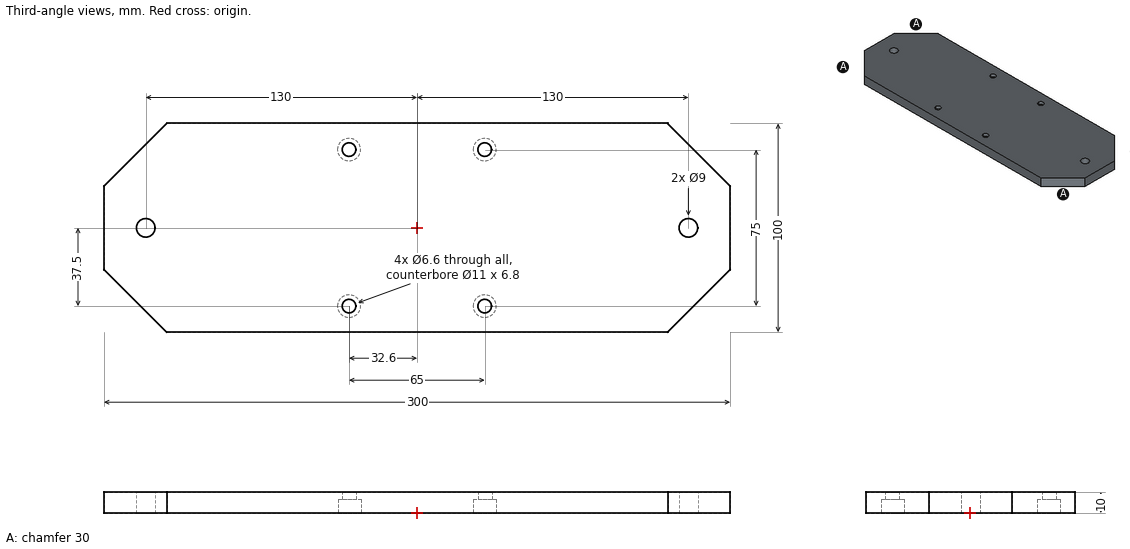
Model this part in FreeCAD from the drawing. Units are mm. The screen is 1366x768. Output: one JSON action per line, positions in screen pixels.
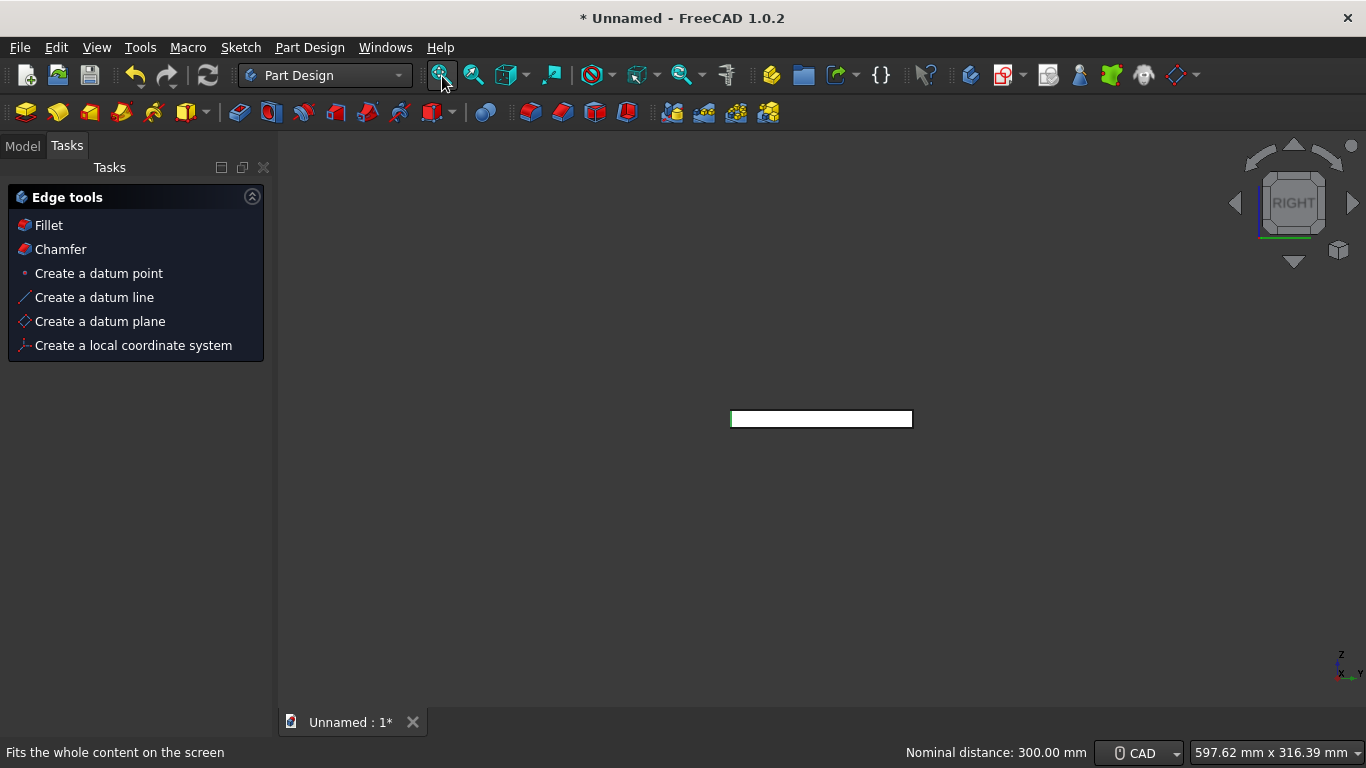
{"action": "left_click", "coordinate": [442, 76]}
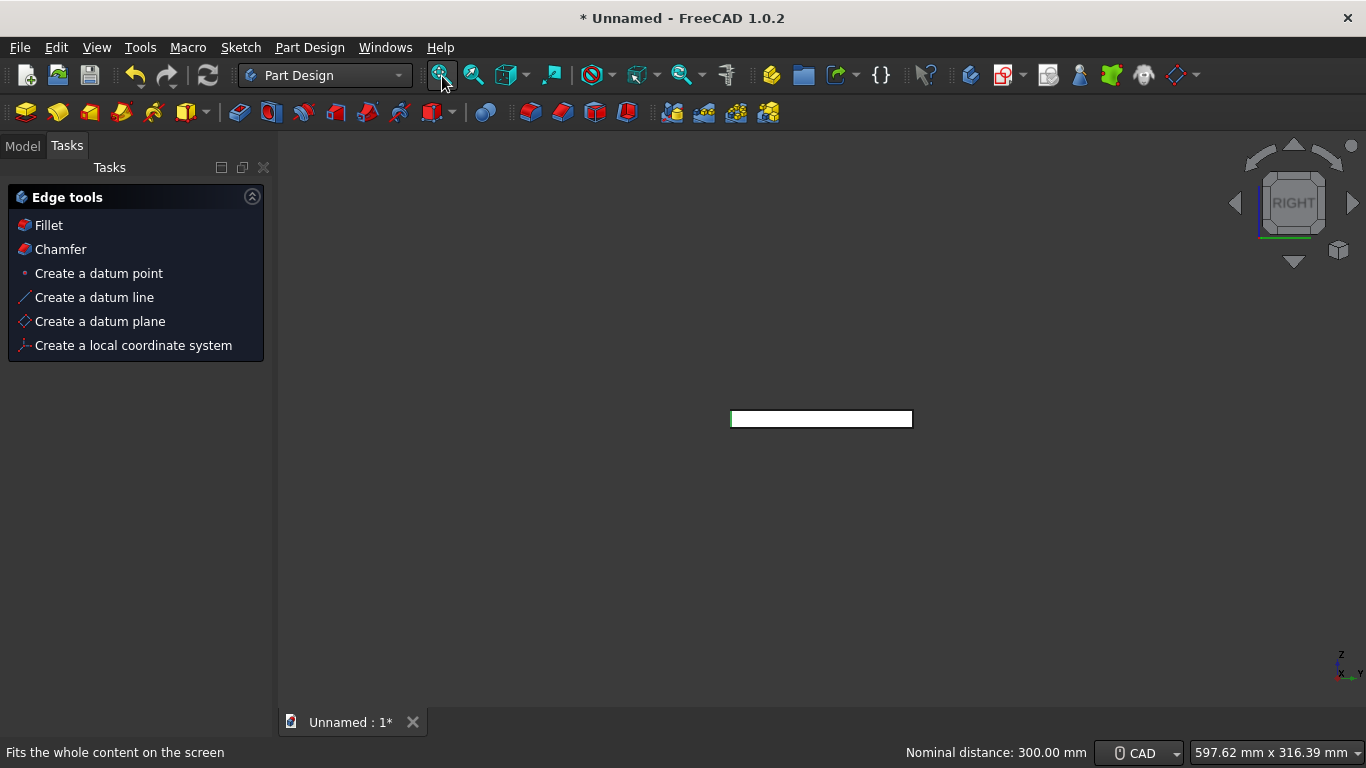
{"action": "left_click", "coordinate": [913, 418], "text": "ctrl"}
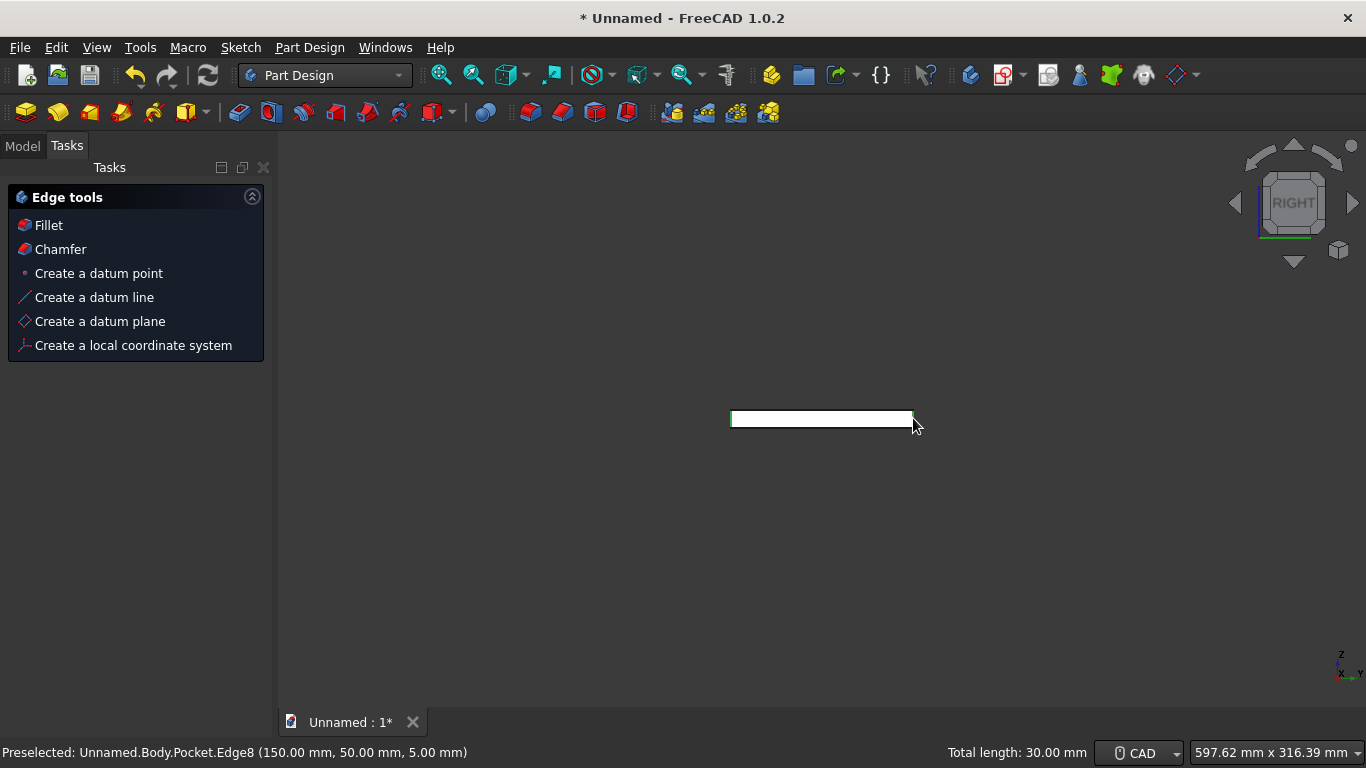
{"action": "scroll", "coordinate": [913, 418], "scroll_direction": "up", "scroll_amount": 4}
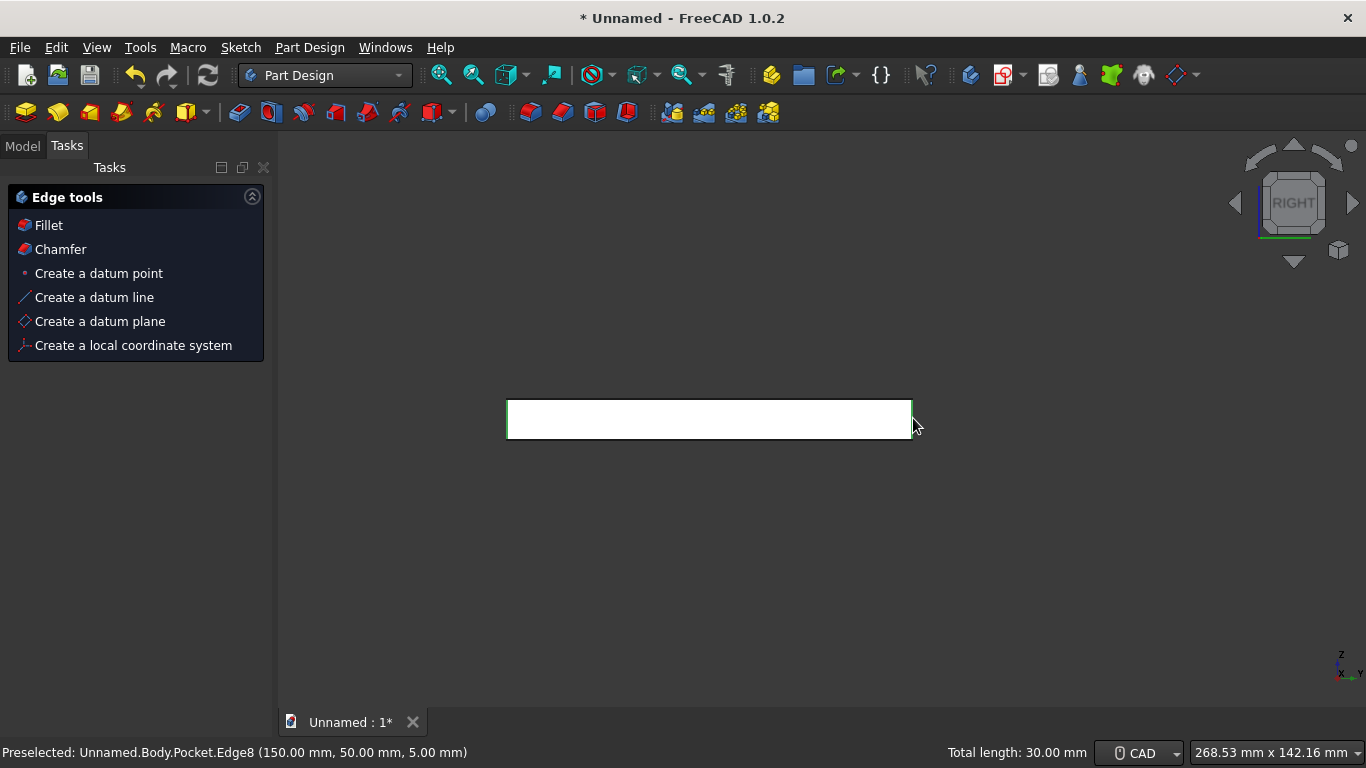
{"action": "left_click", "coordinate": [442, 76]}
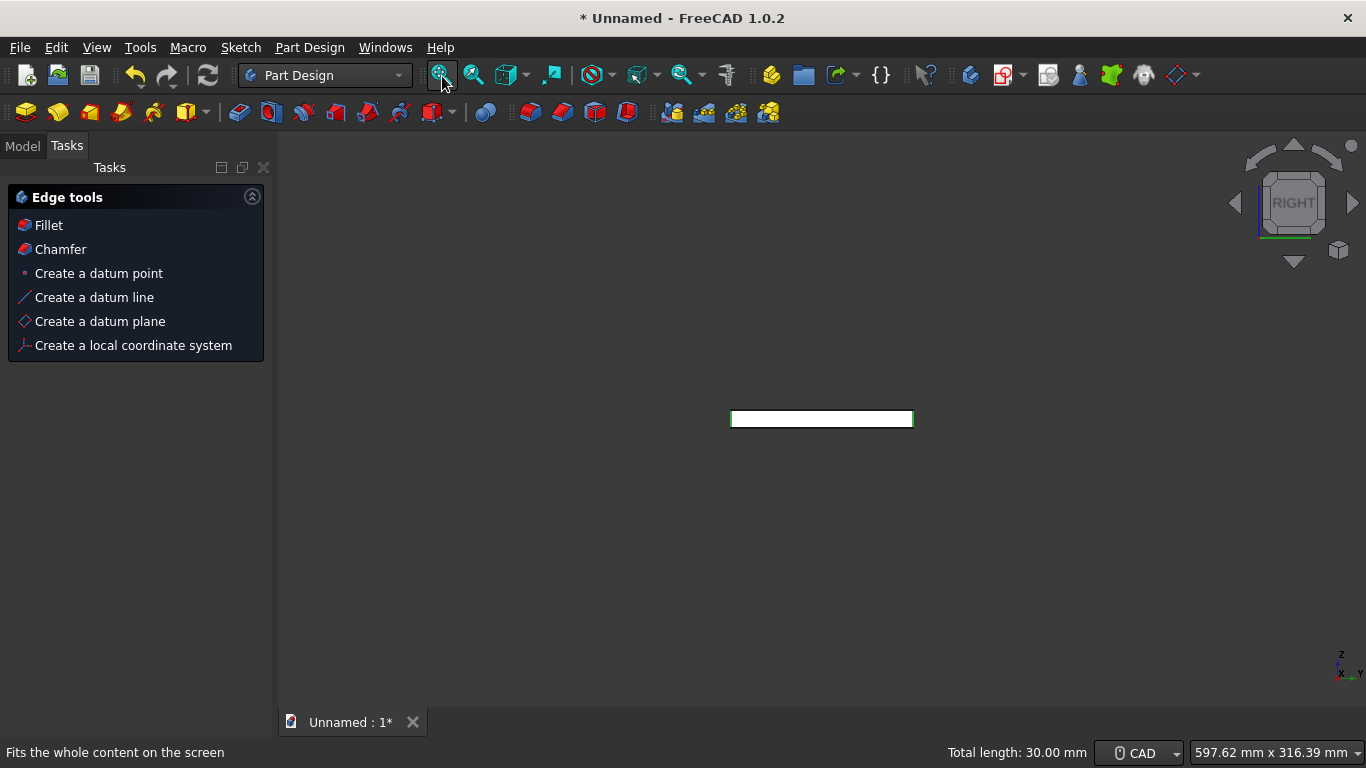
{"action": "key", "text": "5"}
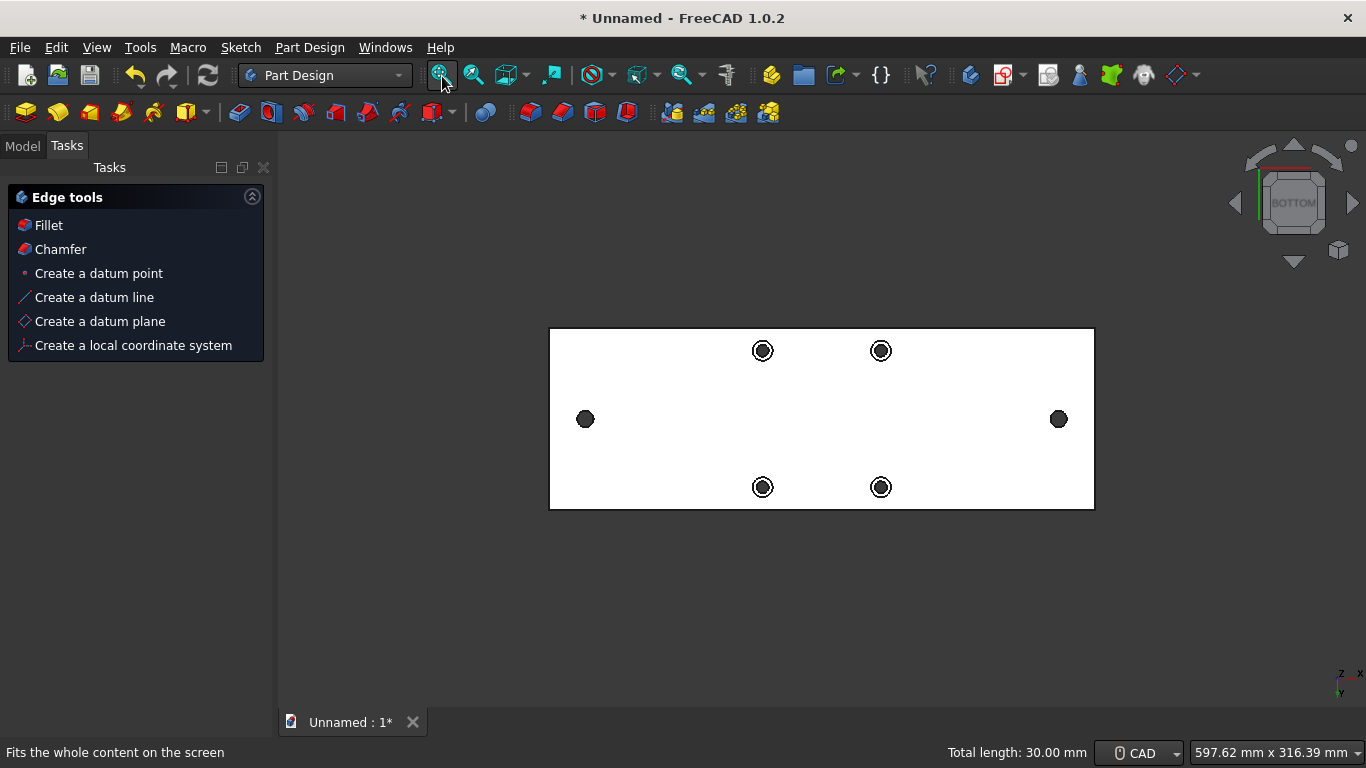
{"action": "scroll", "coordinate": [549, 509], "scroll_direction": "up", "scroll_amount": 4}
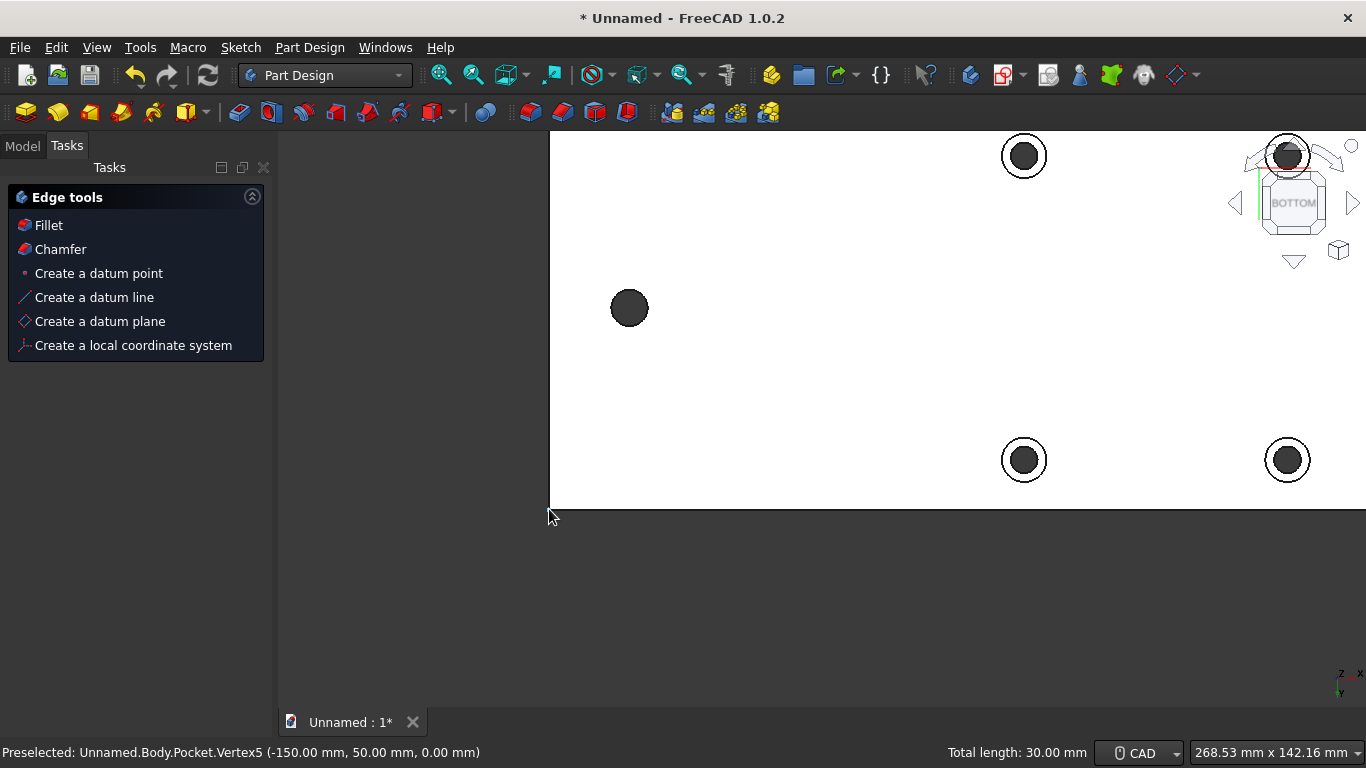
{"action": "key", "text": "v f"}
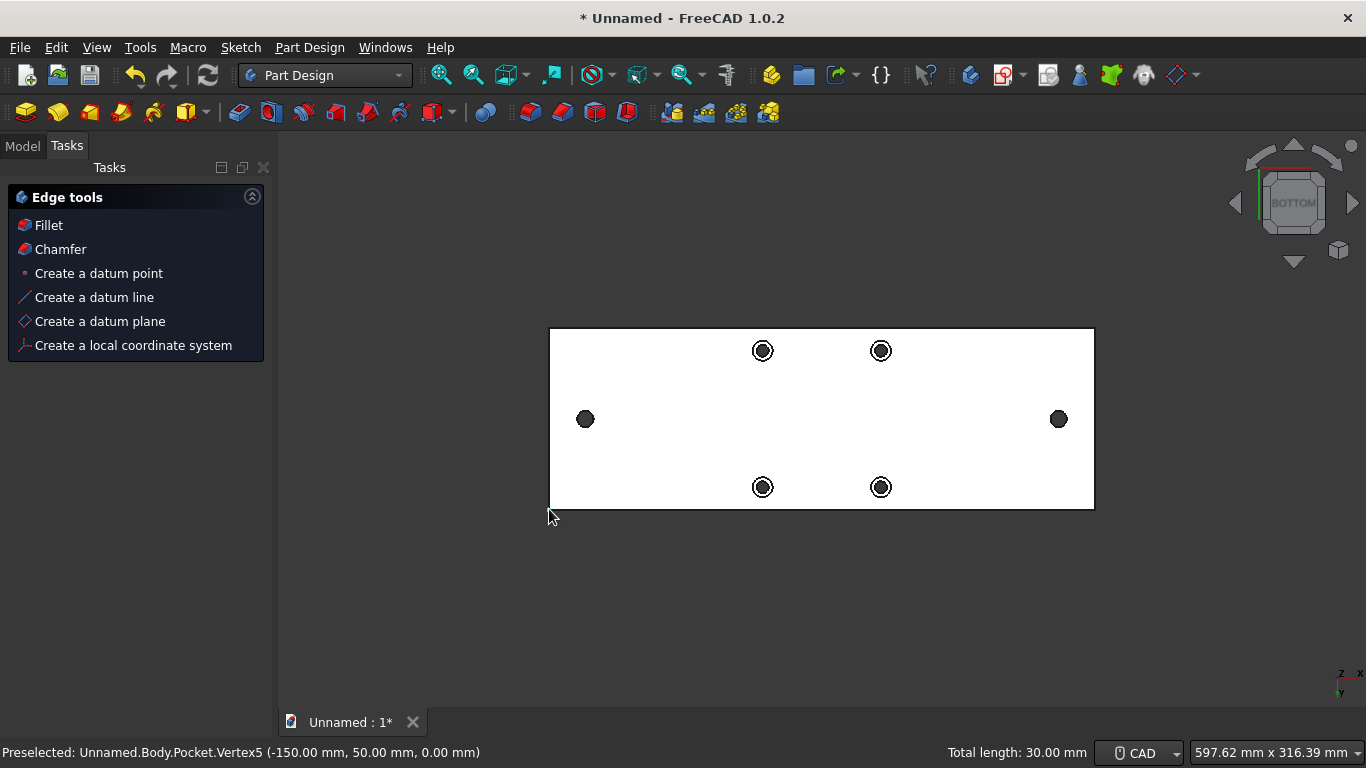
{"action": "key", "text": "4"}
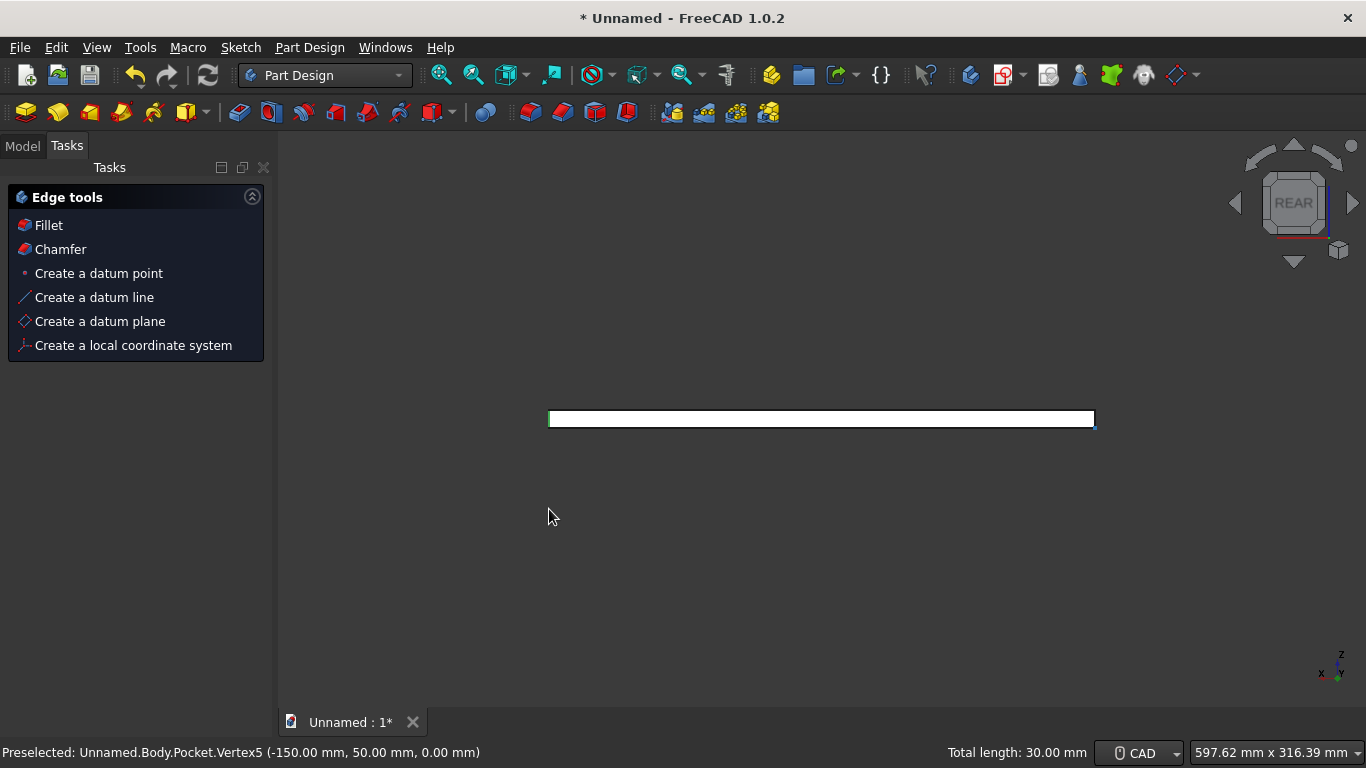
{"action": "left_click", "coordinate": [1095, 418], "text": "ctrl"}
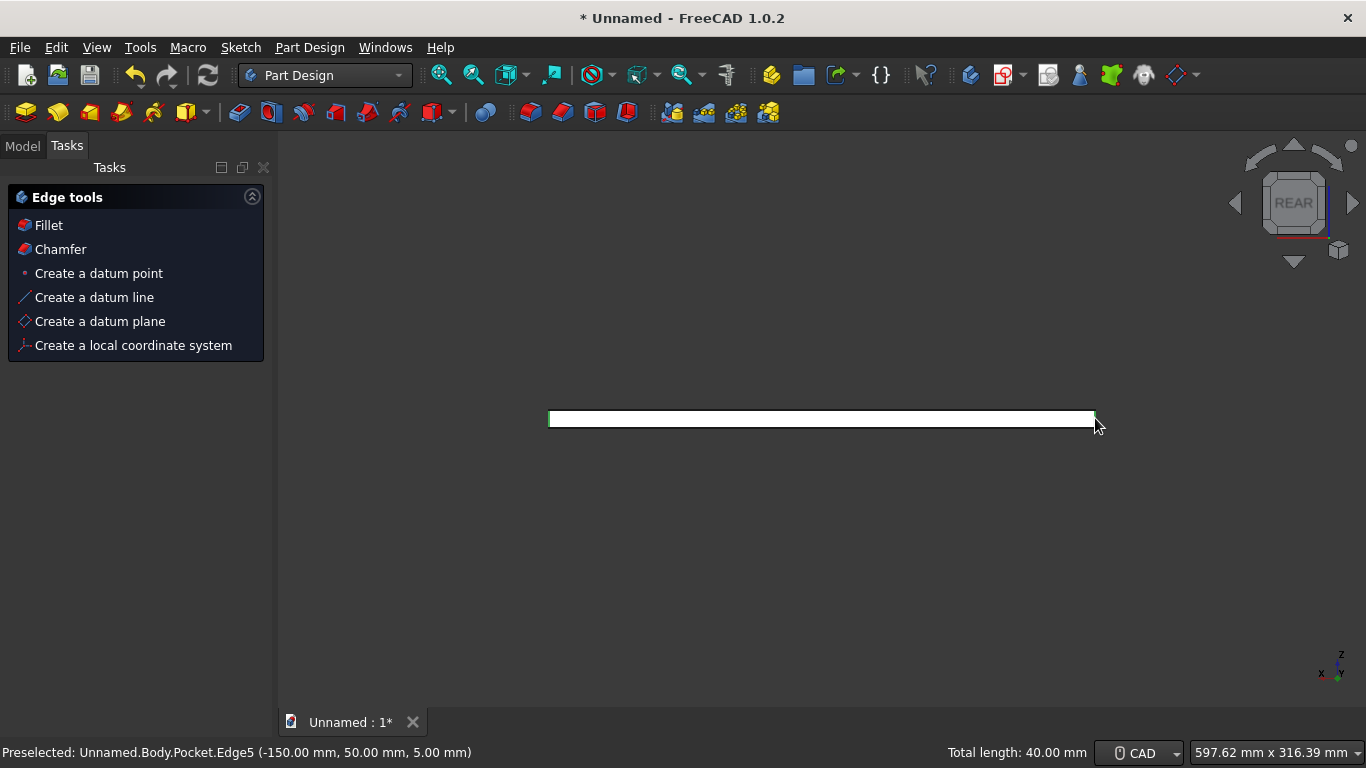
{"action": "left_click", "coordinate": [564, 112]}